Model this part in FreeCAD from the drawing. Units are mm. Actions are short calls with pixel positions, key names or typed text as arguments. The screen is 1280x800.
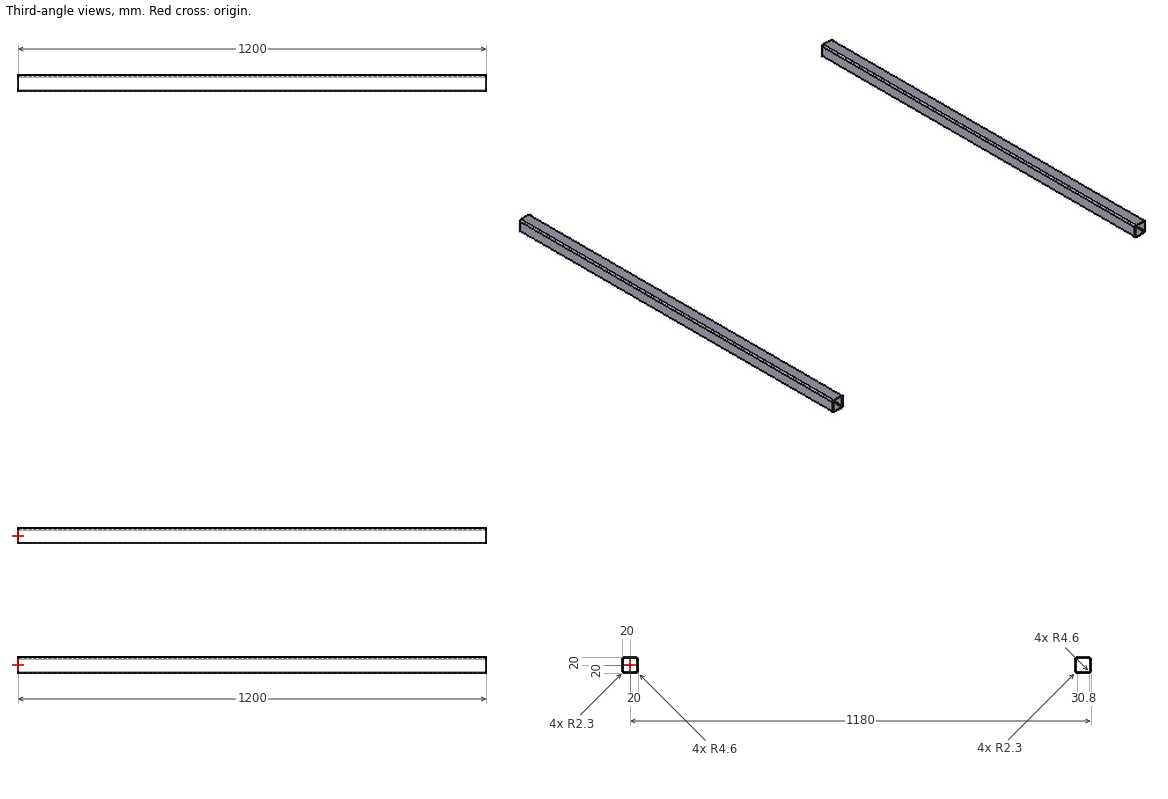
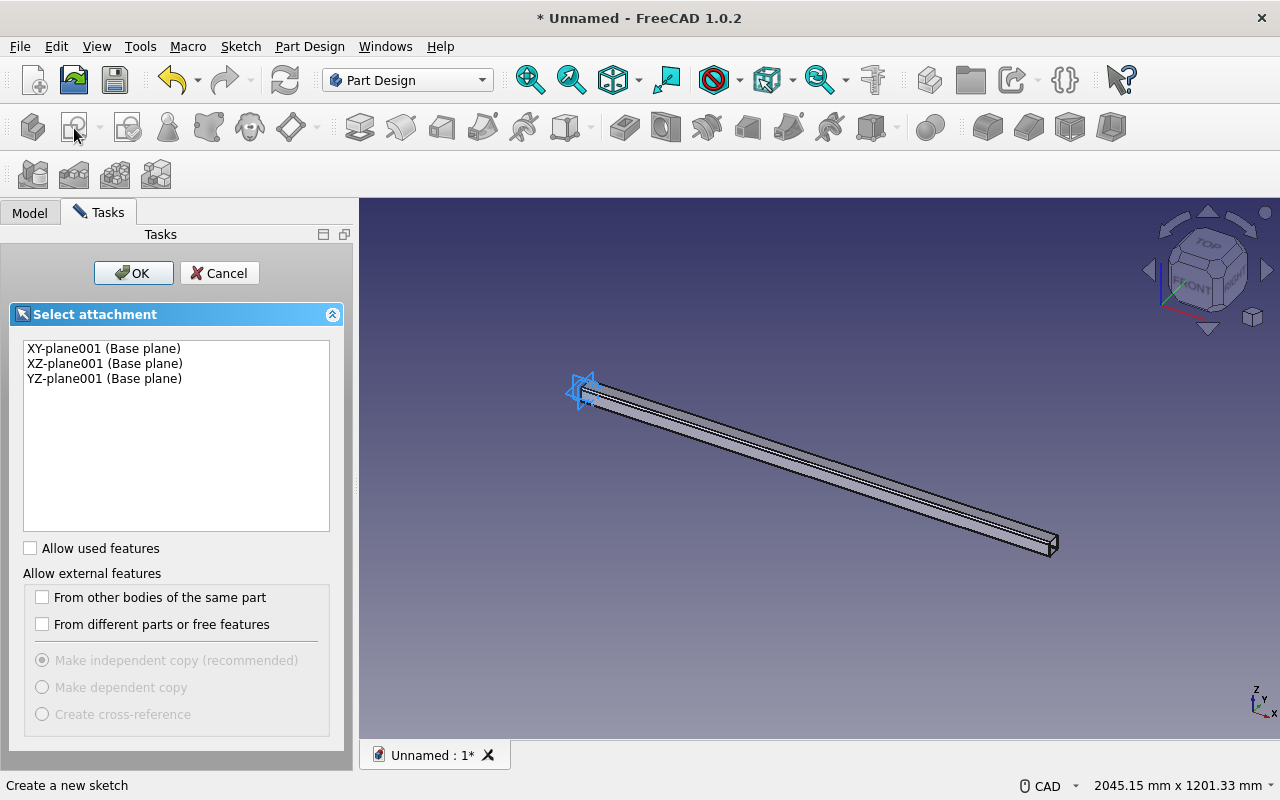
click(84, 378)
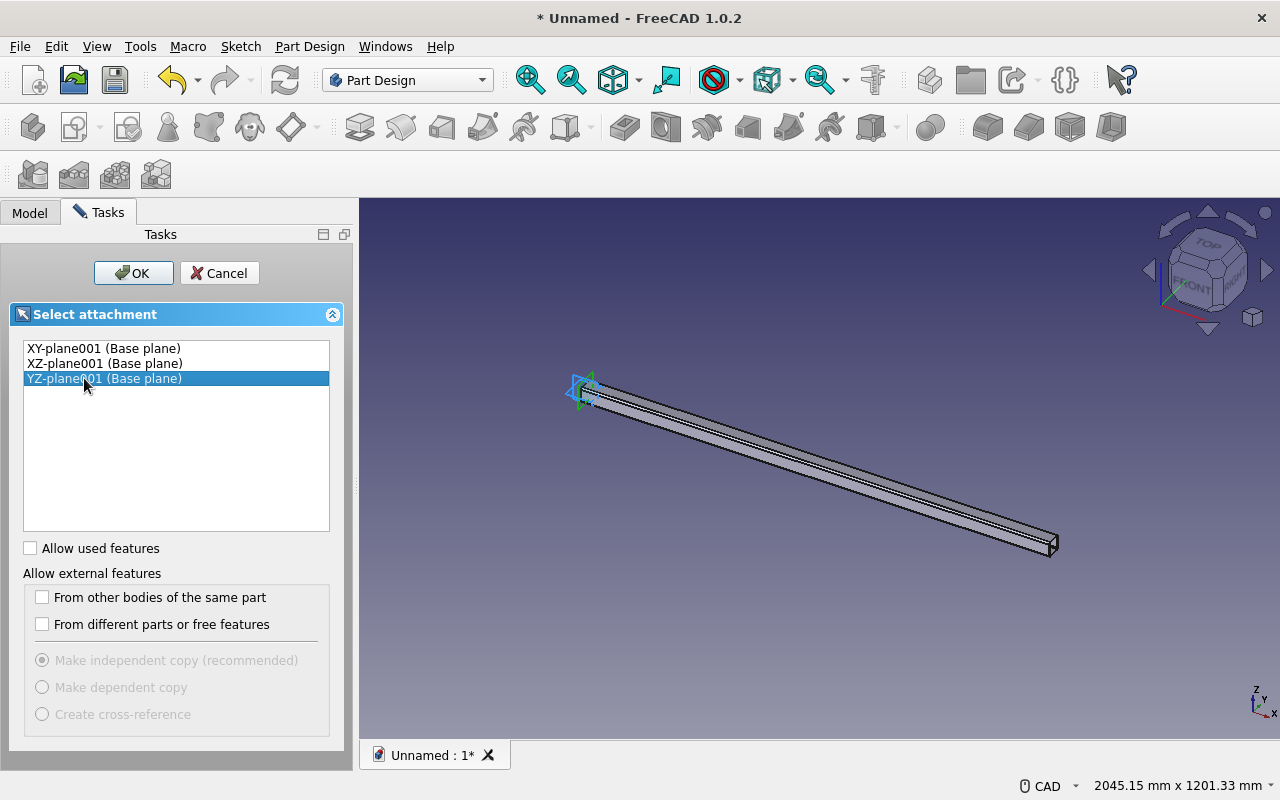
click(134, 273)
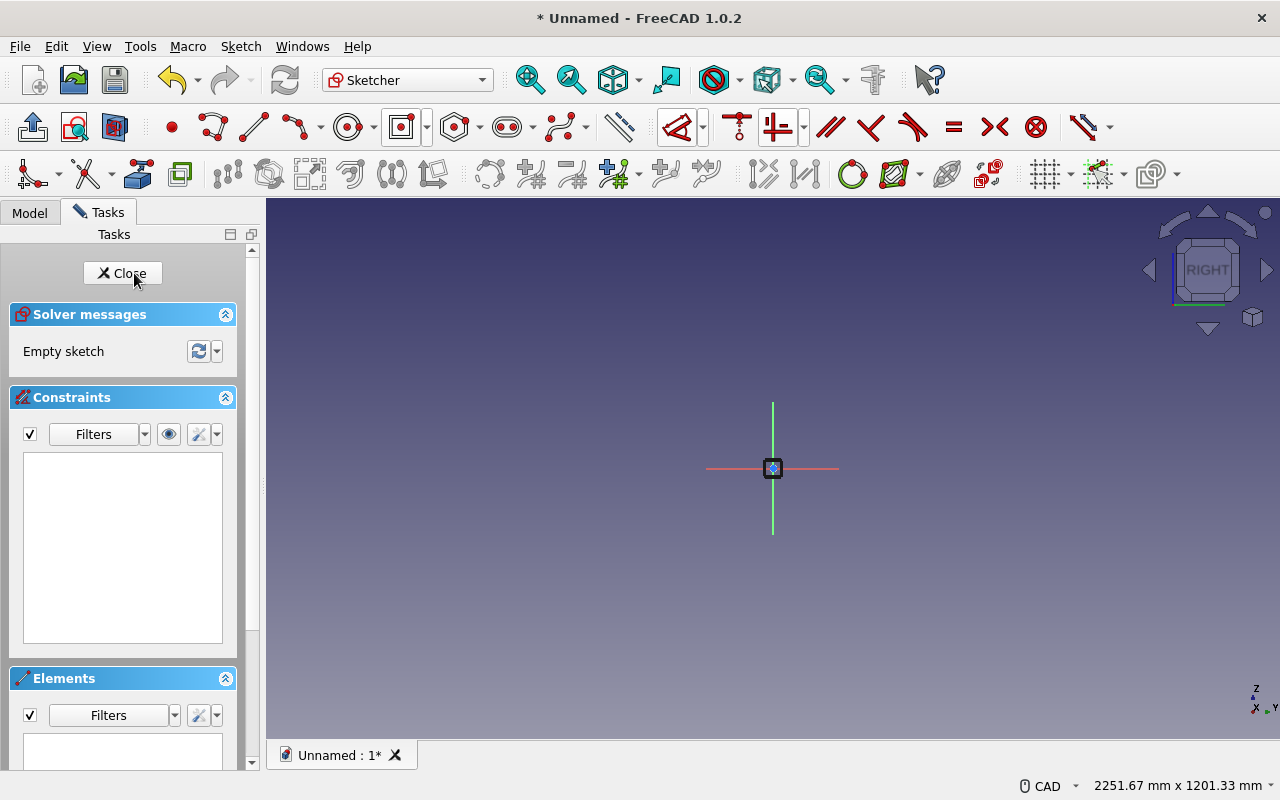
scroll(704, 468, down, 5)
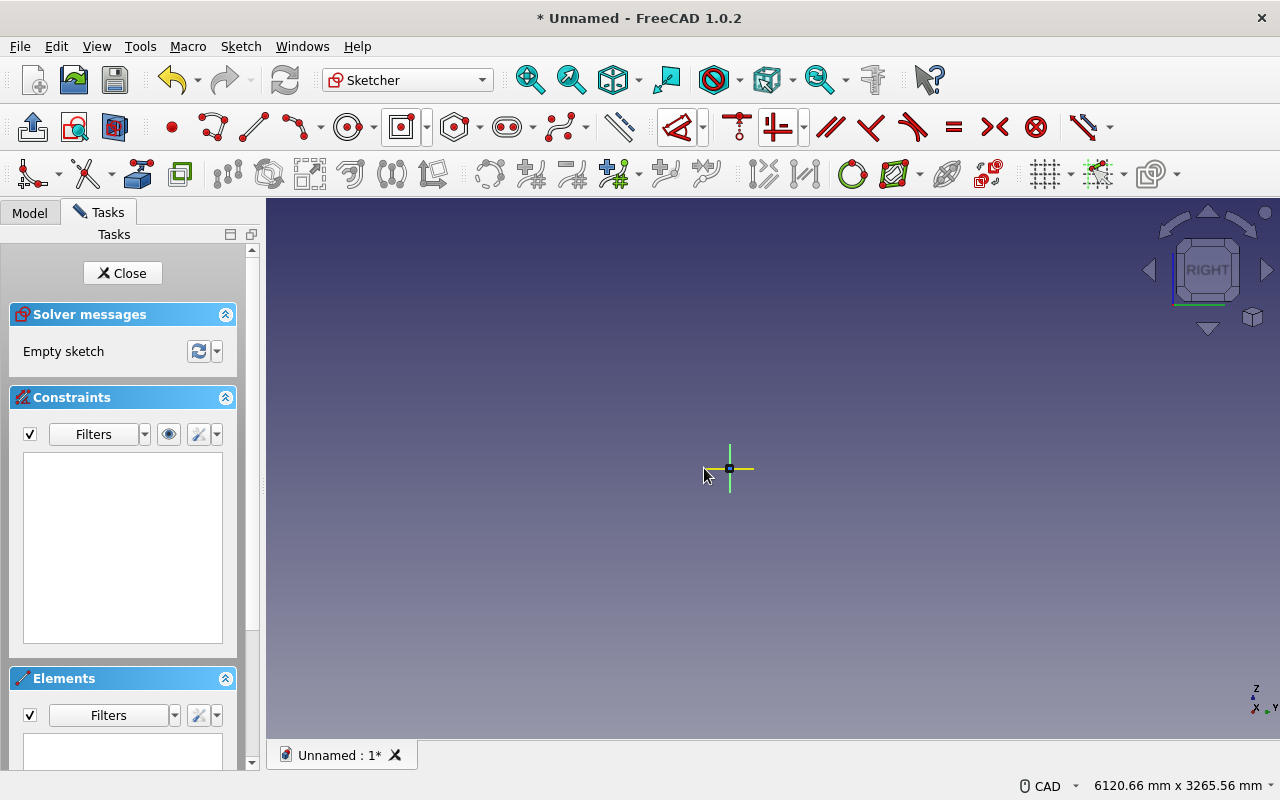
scroll(933, 468, up, 15)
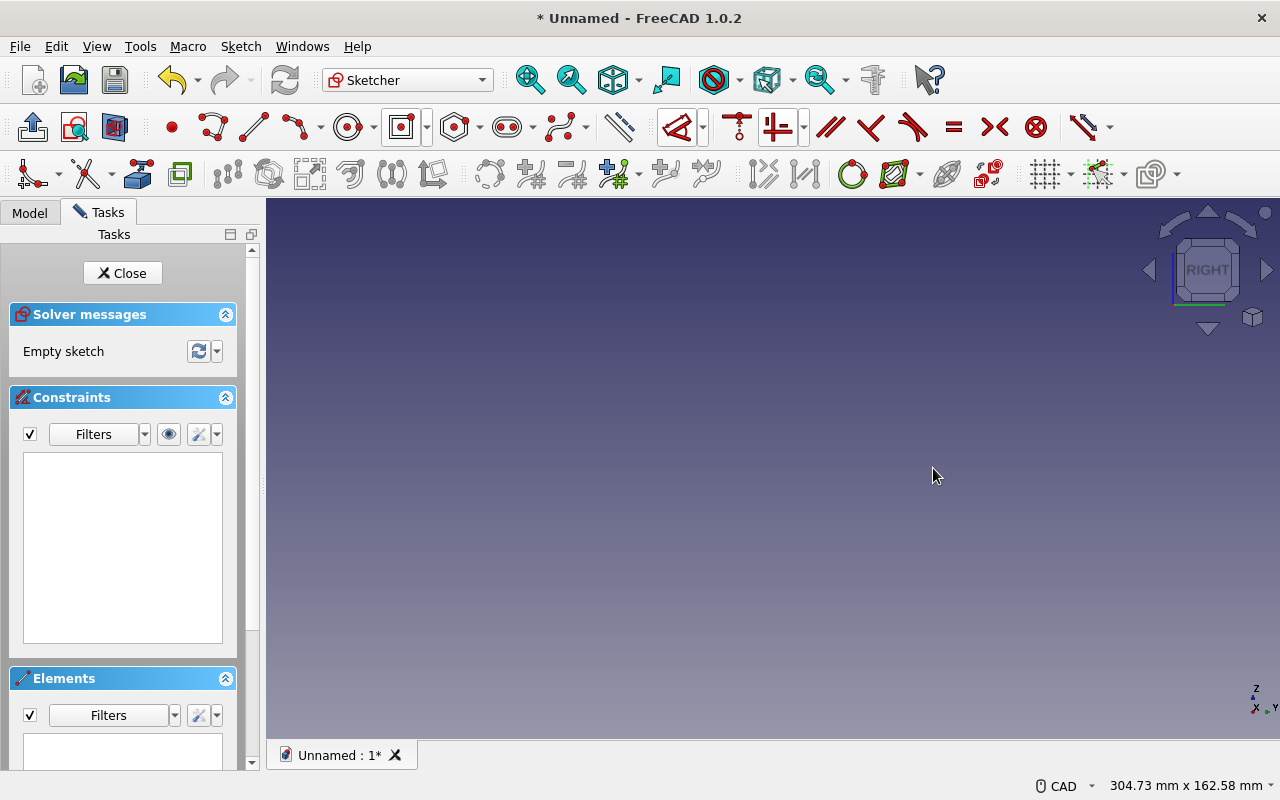
scroll(691, 468, up, 5)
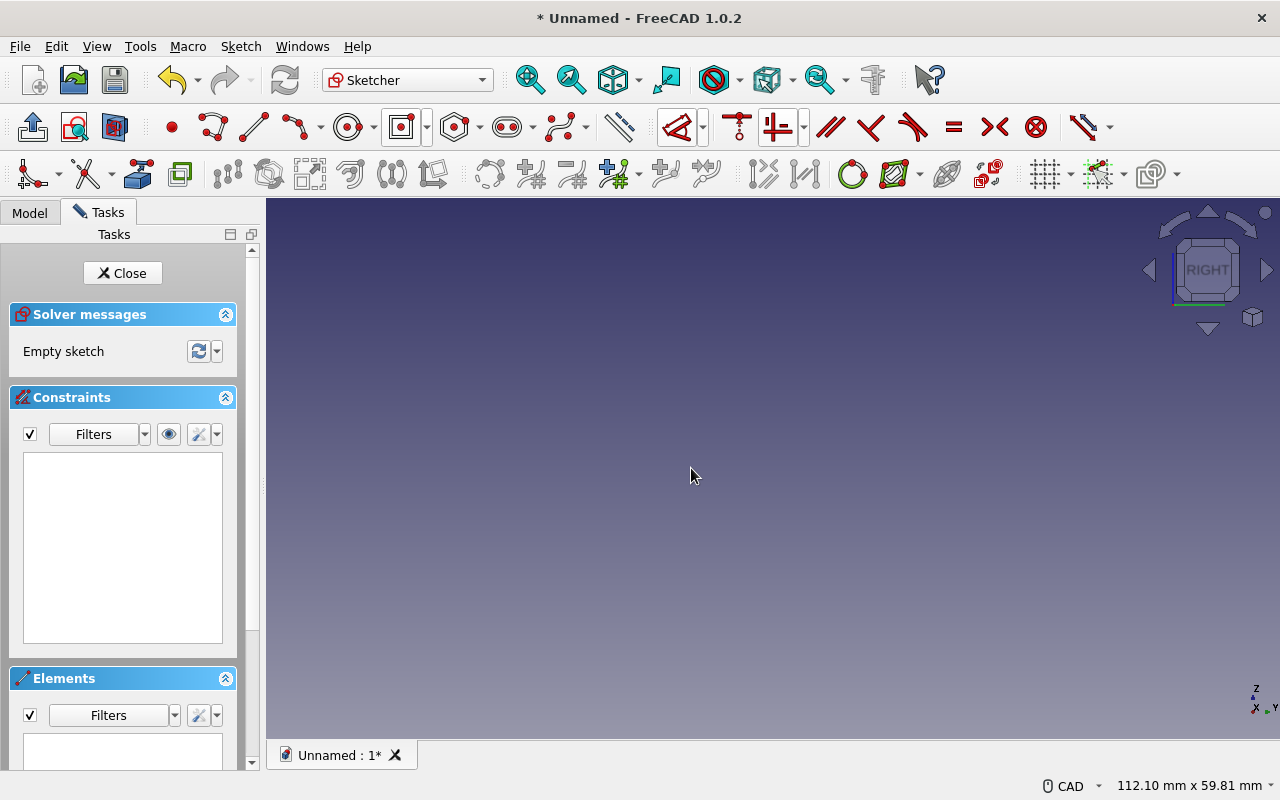
key(g)
key(l)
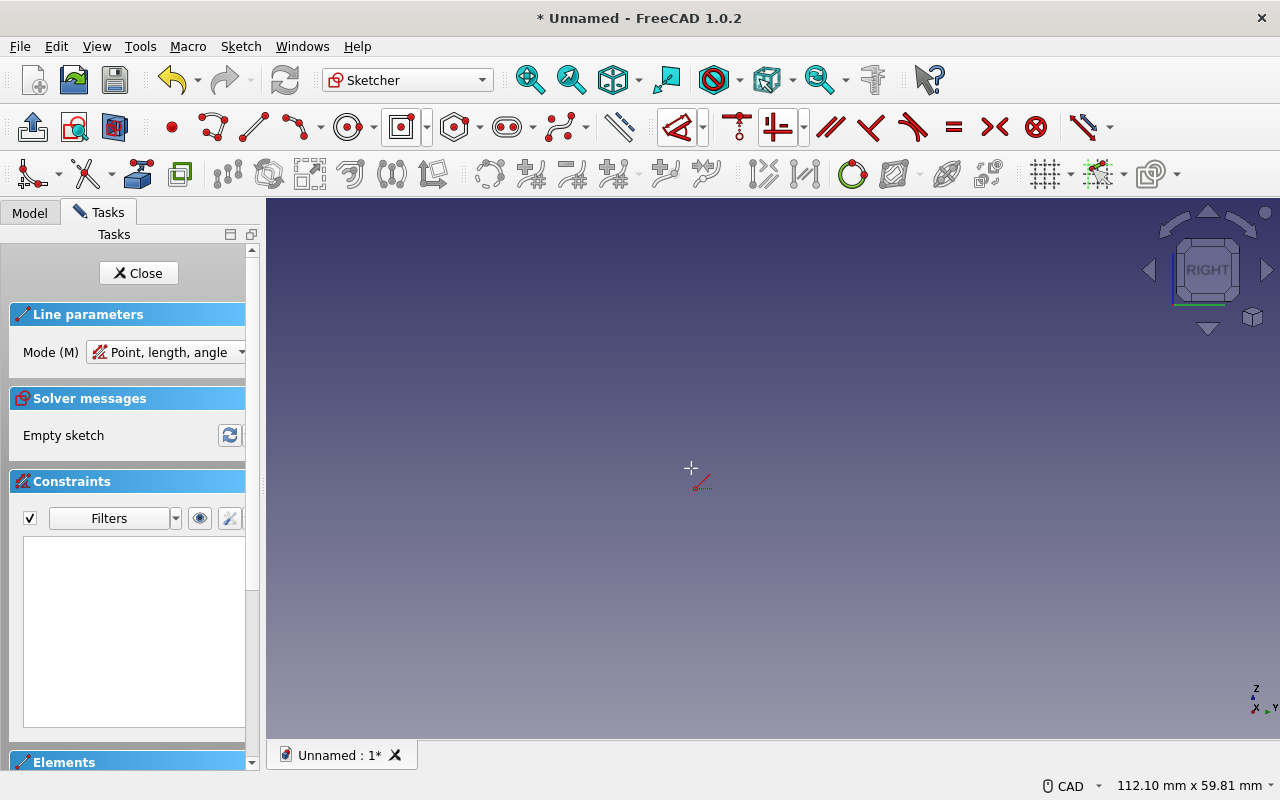
click(565, 649)
click(843, 649)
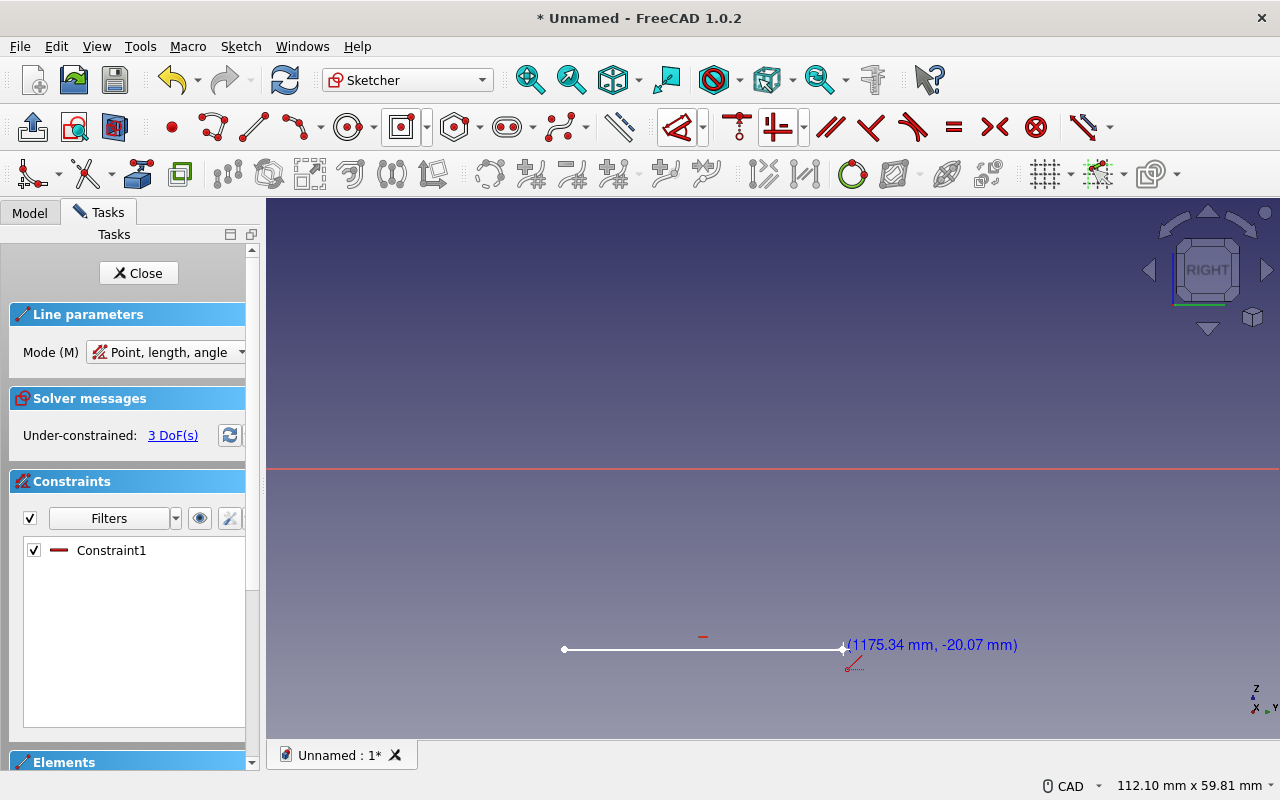
click(885, 608)
click(885, 329)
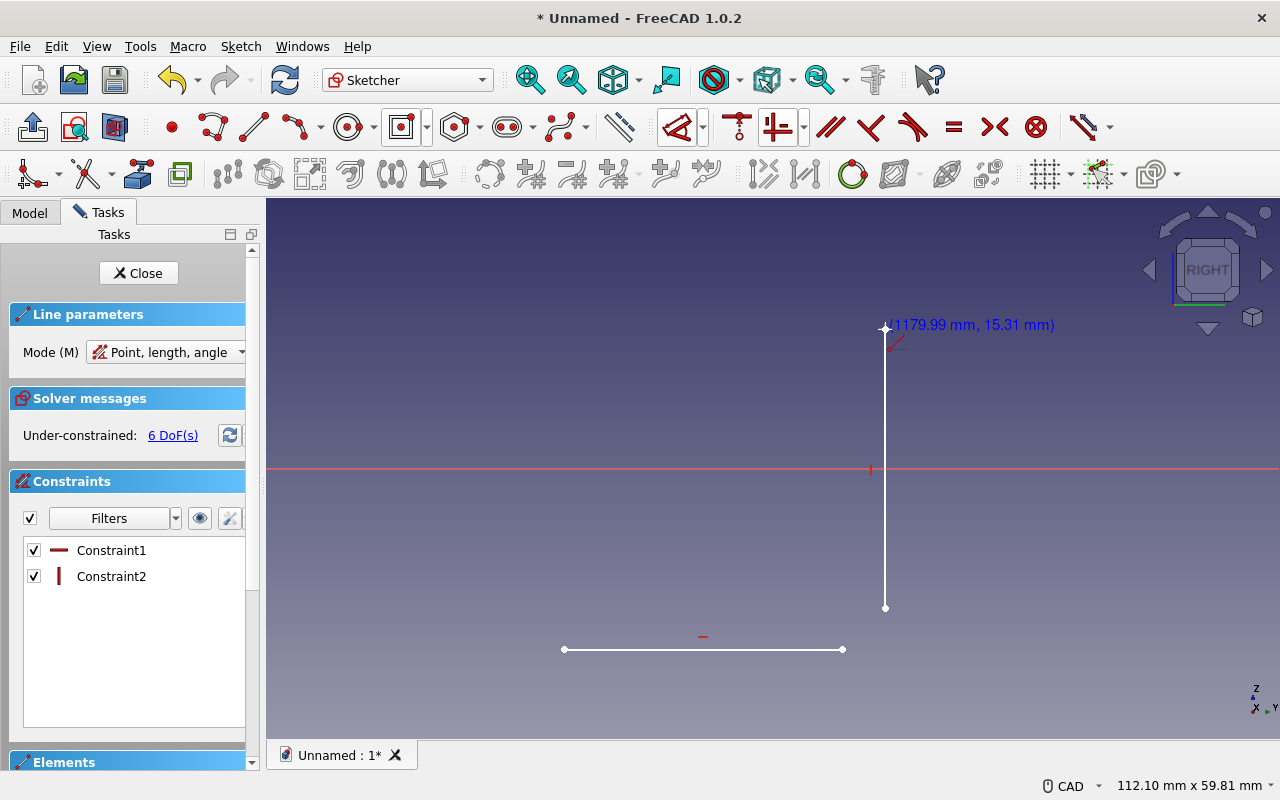
click(843, 288)
click(565, 288)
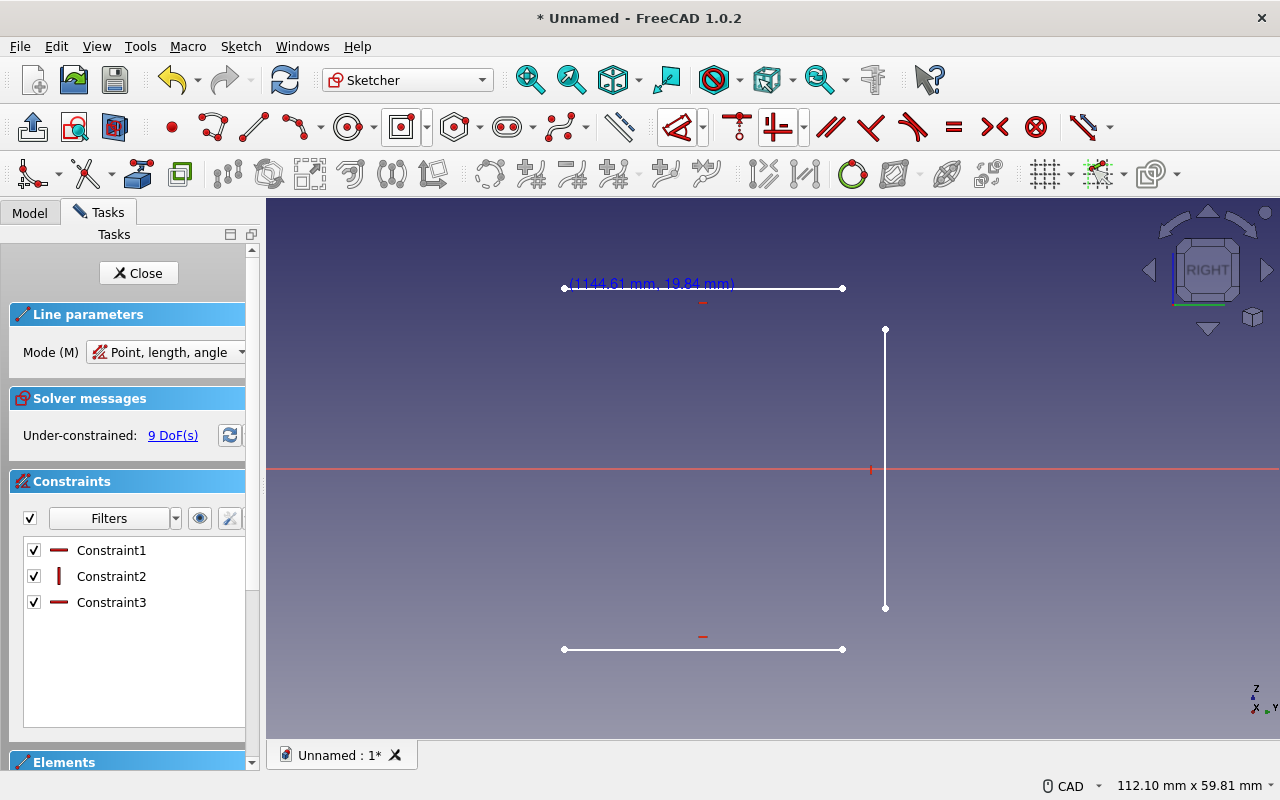
click(523, 329)
click(523, 608)